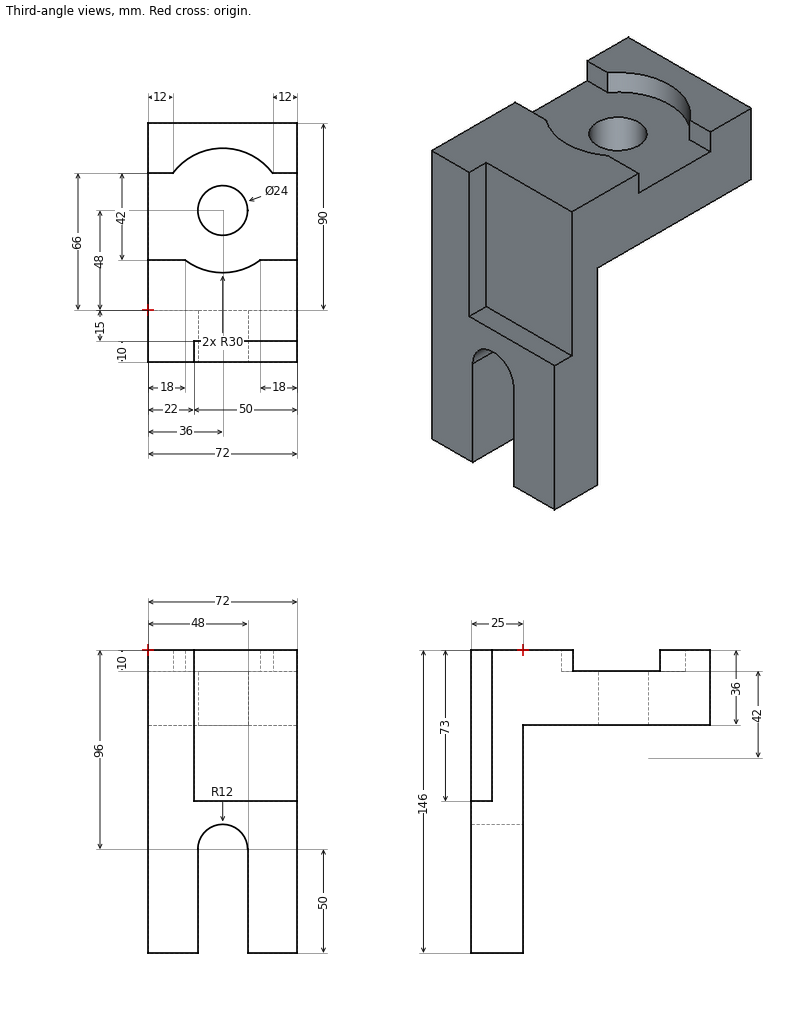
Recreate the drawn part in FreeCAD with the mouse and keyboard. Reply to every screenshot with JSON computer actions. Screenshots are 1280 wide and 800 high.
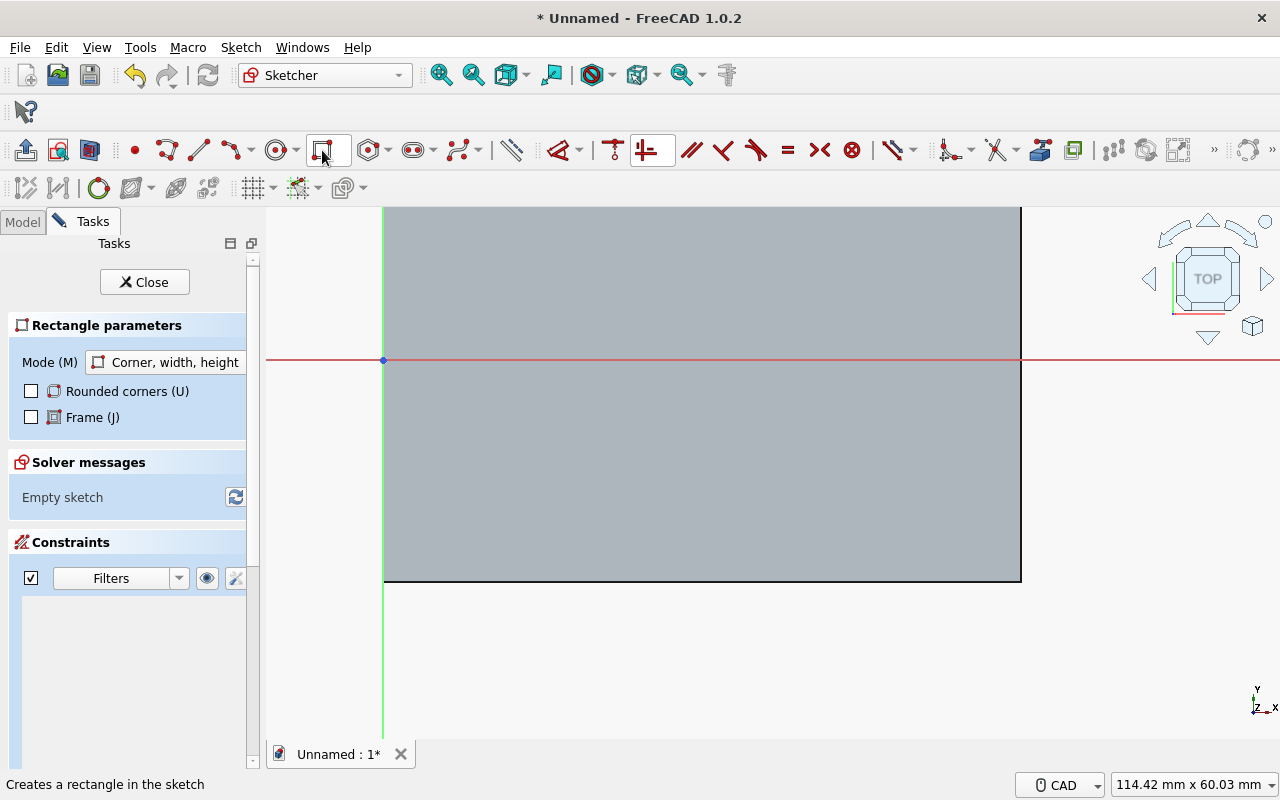
{"action": "left_click", "coordinate": [578, 493]}
{"action": "left_click", "coordinate": [1021, 582]}
{"action": "key", "text": "Escape"}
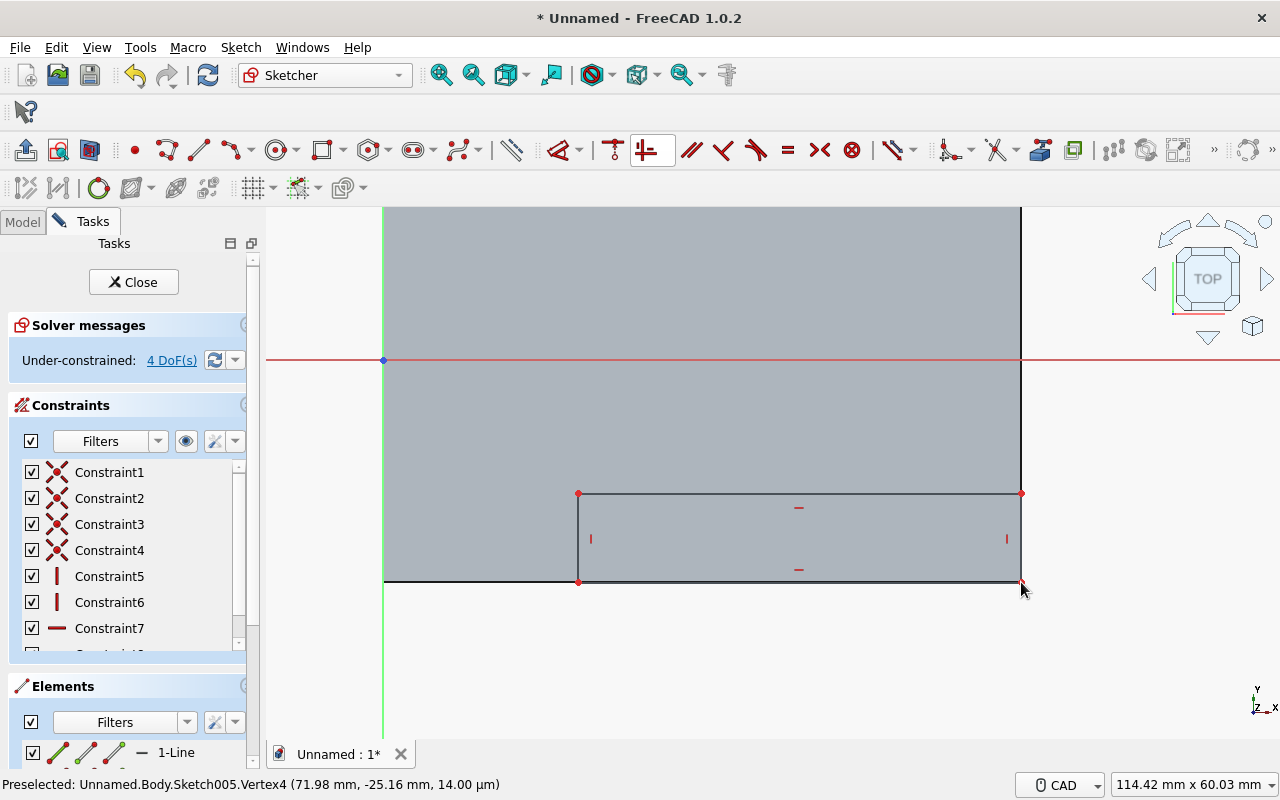
{"action": "left_click", "coordinate": [558, 150]}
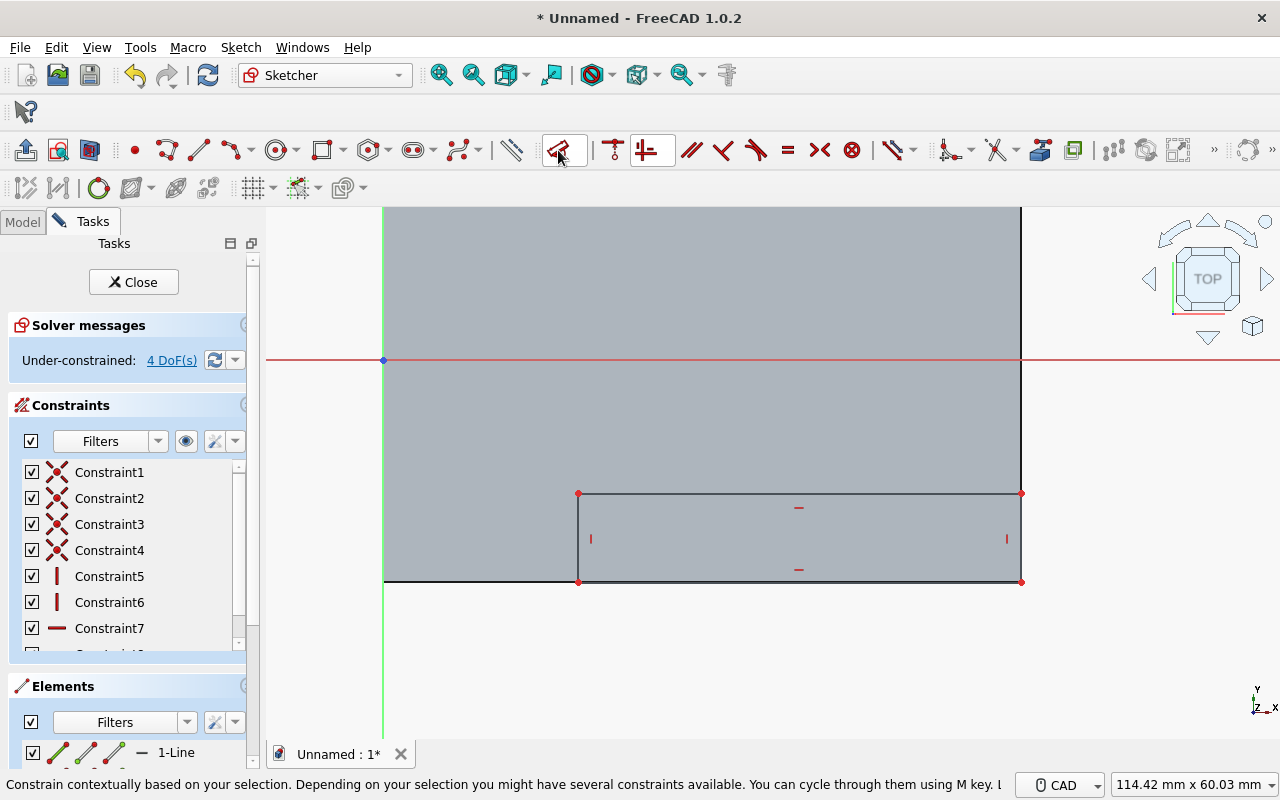
{"action": "left_click", "coordinate": [578, 521]}
{"action": "left_click", "coordinate": [544, 538]}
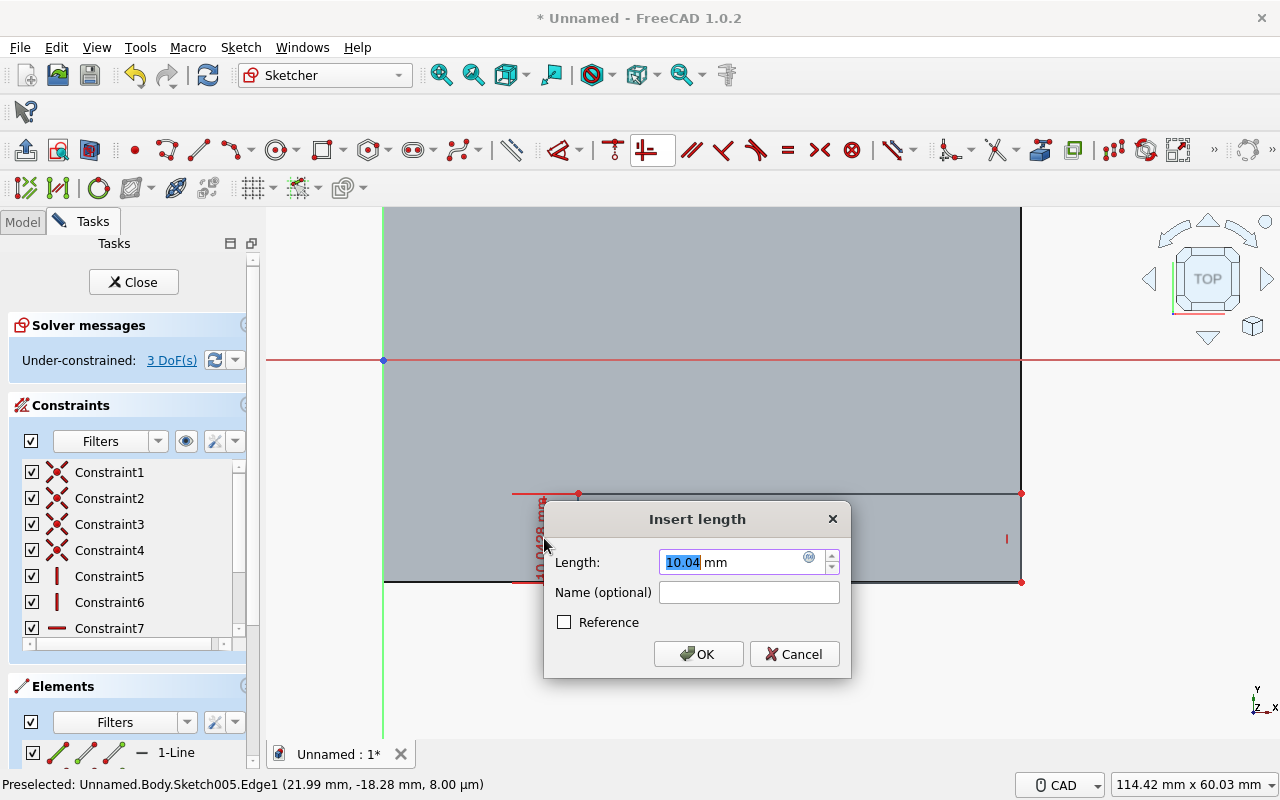
{"action": "type", "text": "10"}
{"action": "key", "text": "Return"}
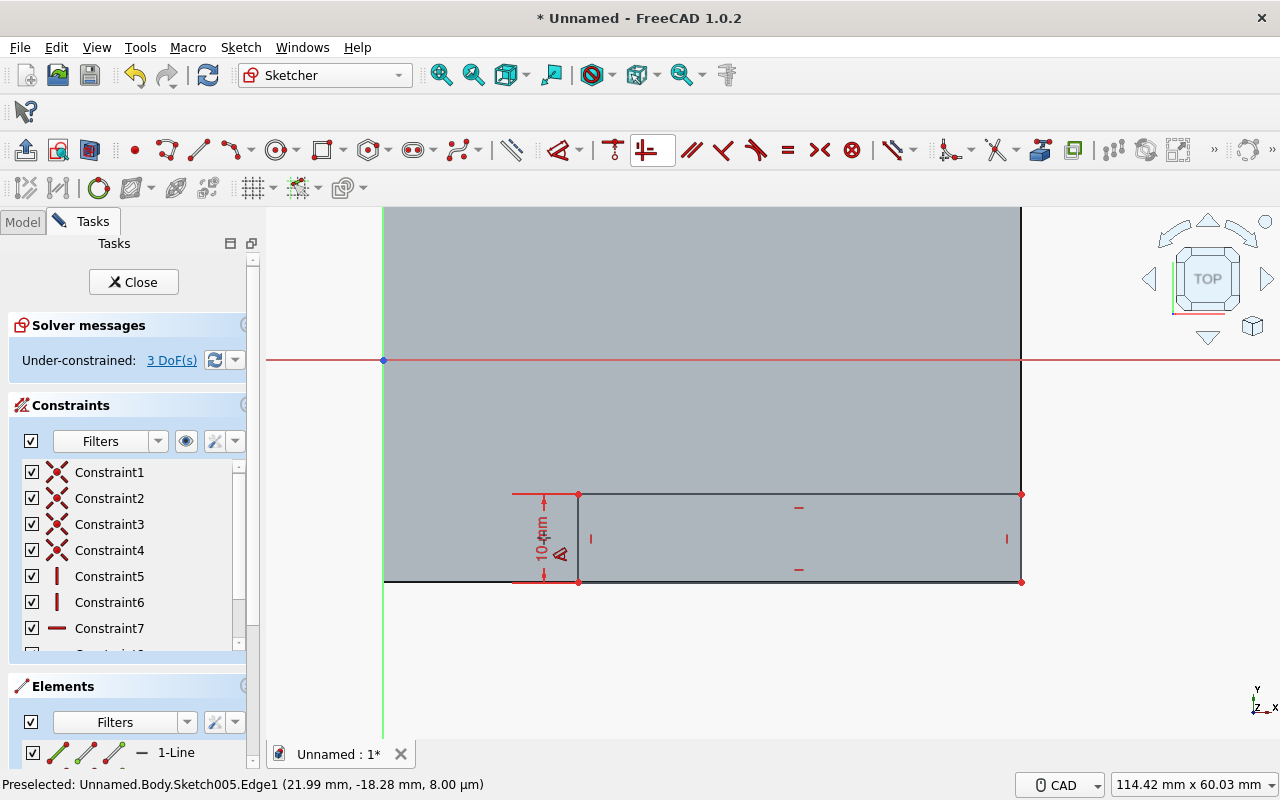
{"action": "left_click", "coordinate": [711, 583]}
{"action": "left_click", "coordinate": [799, 617]}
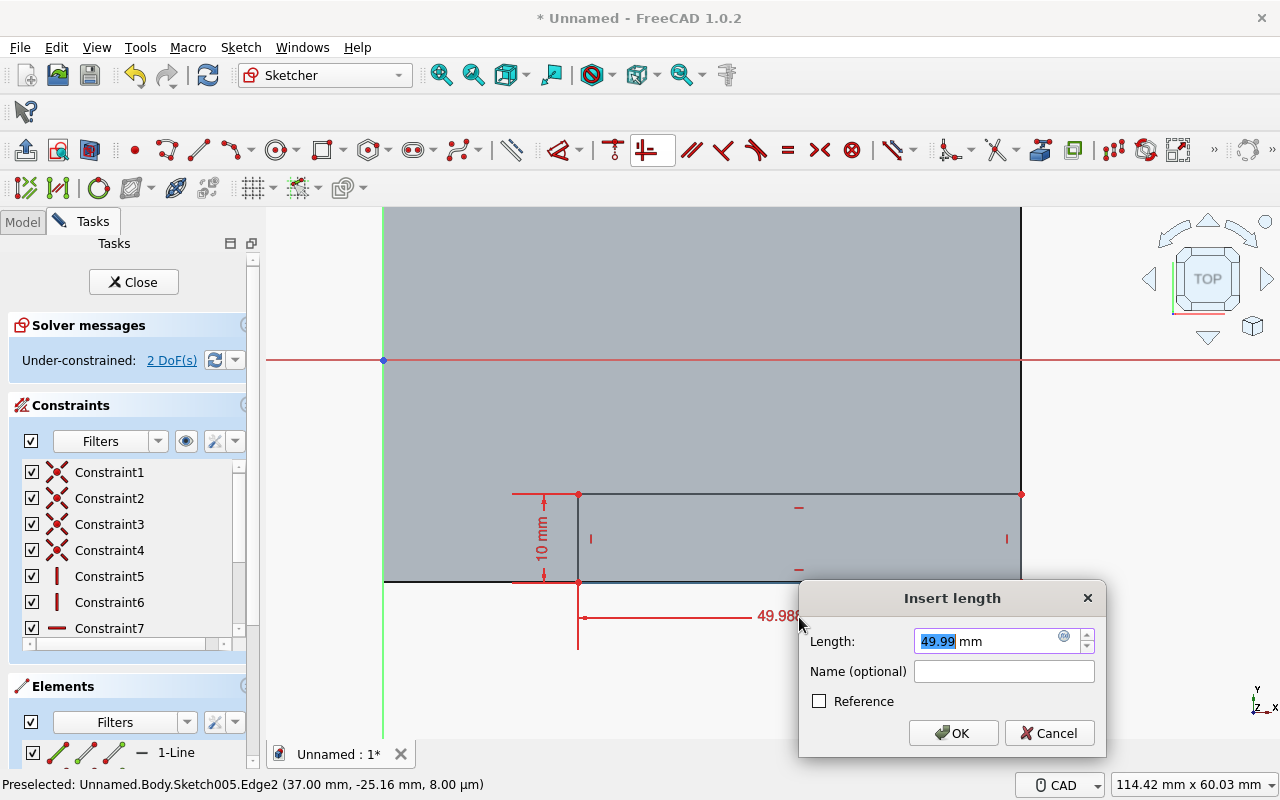
{"action": "type", "text": "50"}
{"action": "key", "text": "Return"}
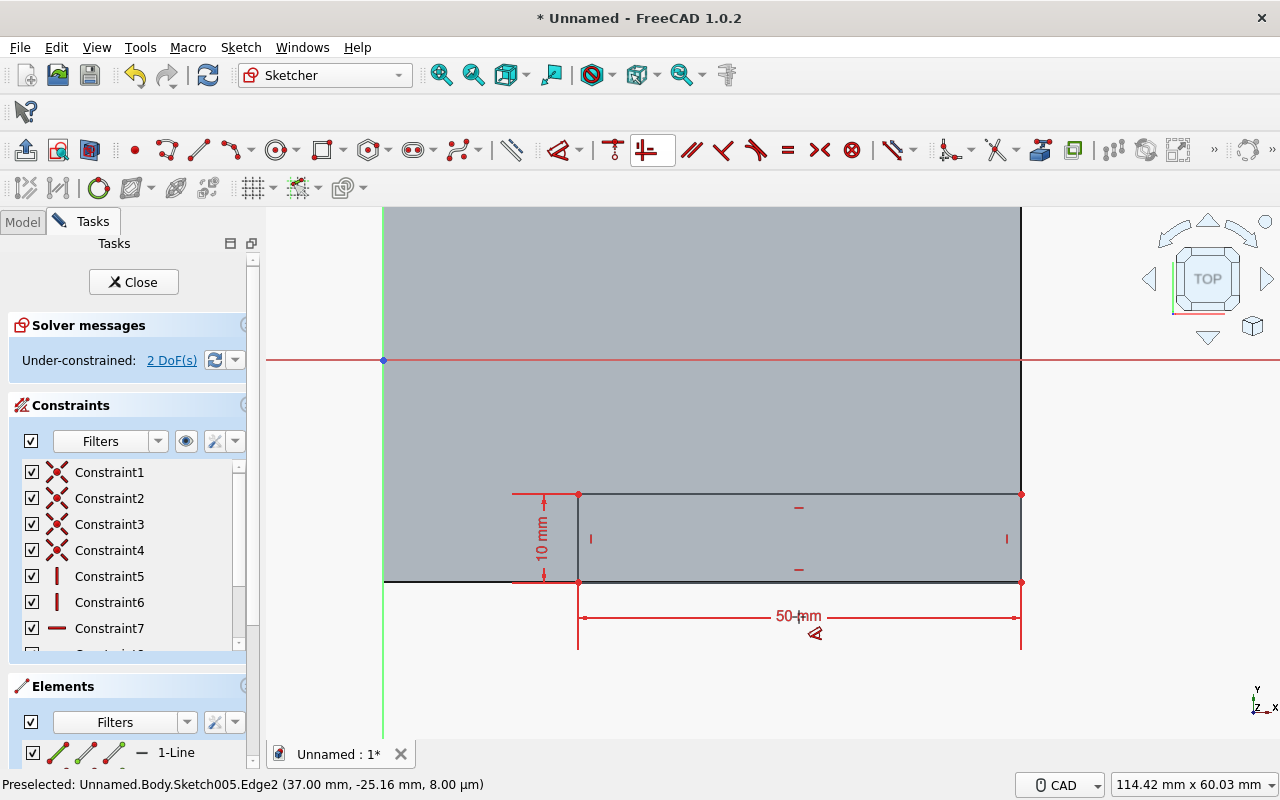
{"action": "left_click", "coordinate": [578, 494]}
{"action": "left_click", "coordinate": [481, 326]}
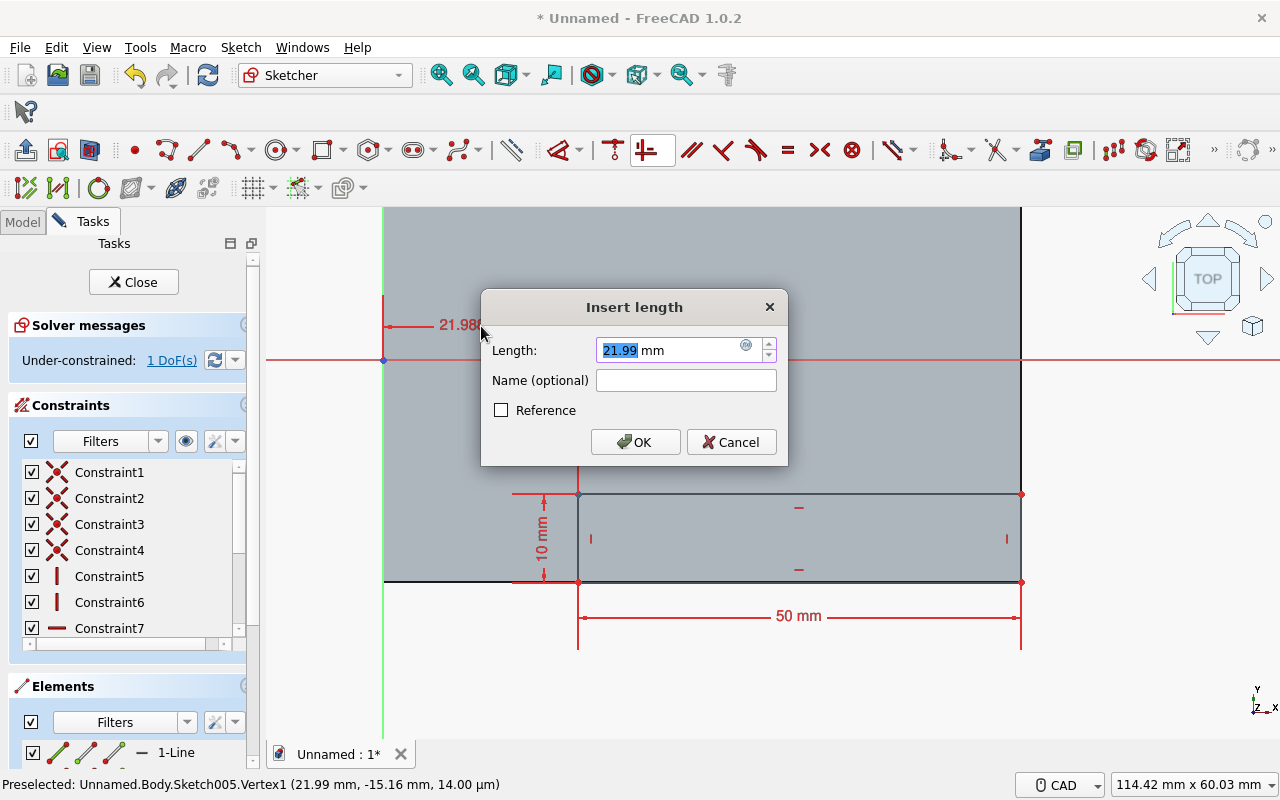
{"action": "type", "text": "22"}
{"action": "key", "text": "Return"}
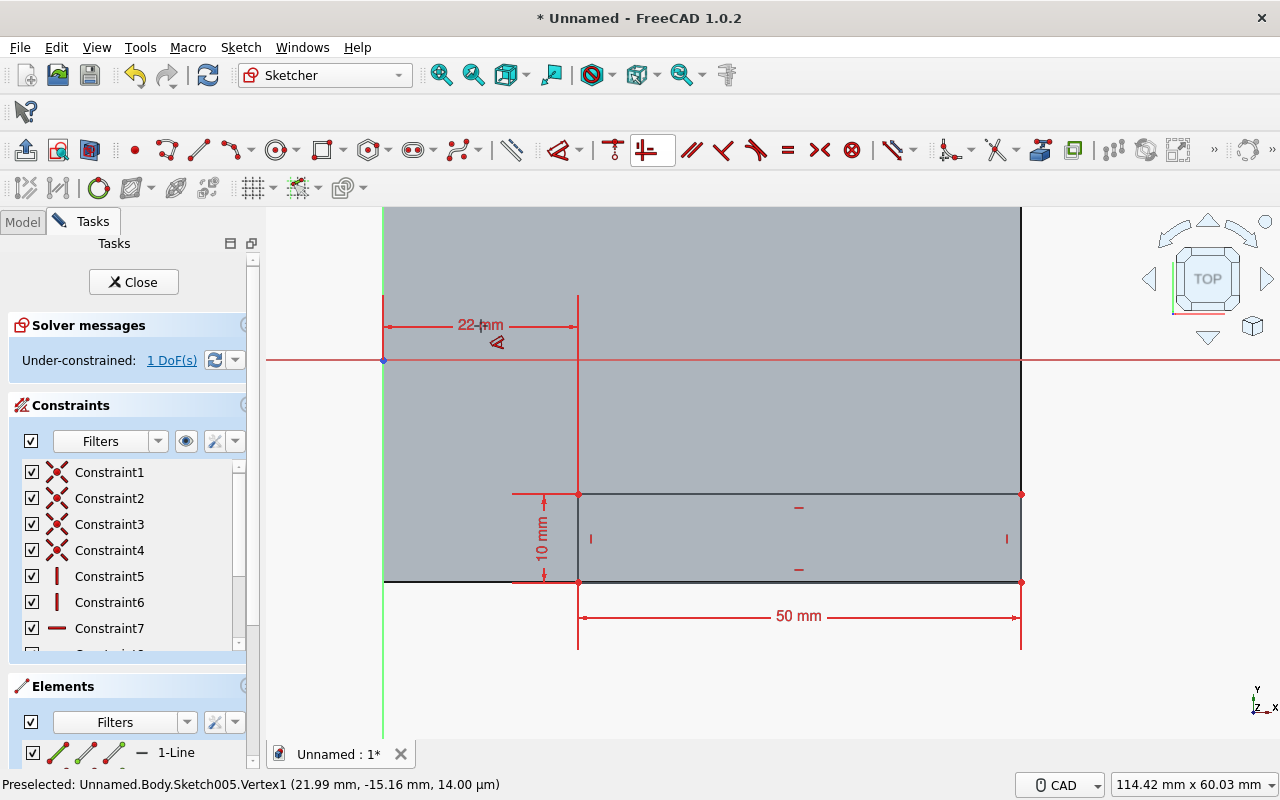
{"action": "left_click", "coordinate": [578, 494]}
{"action": "left_click", "coordinate": [349, 427]}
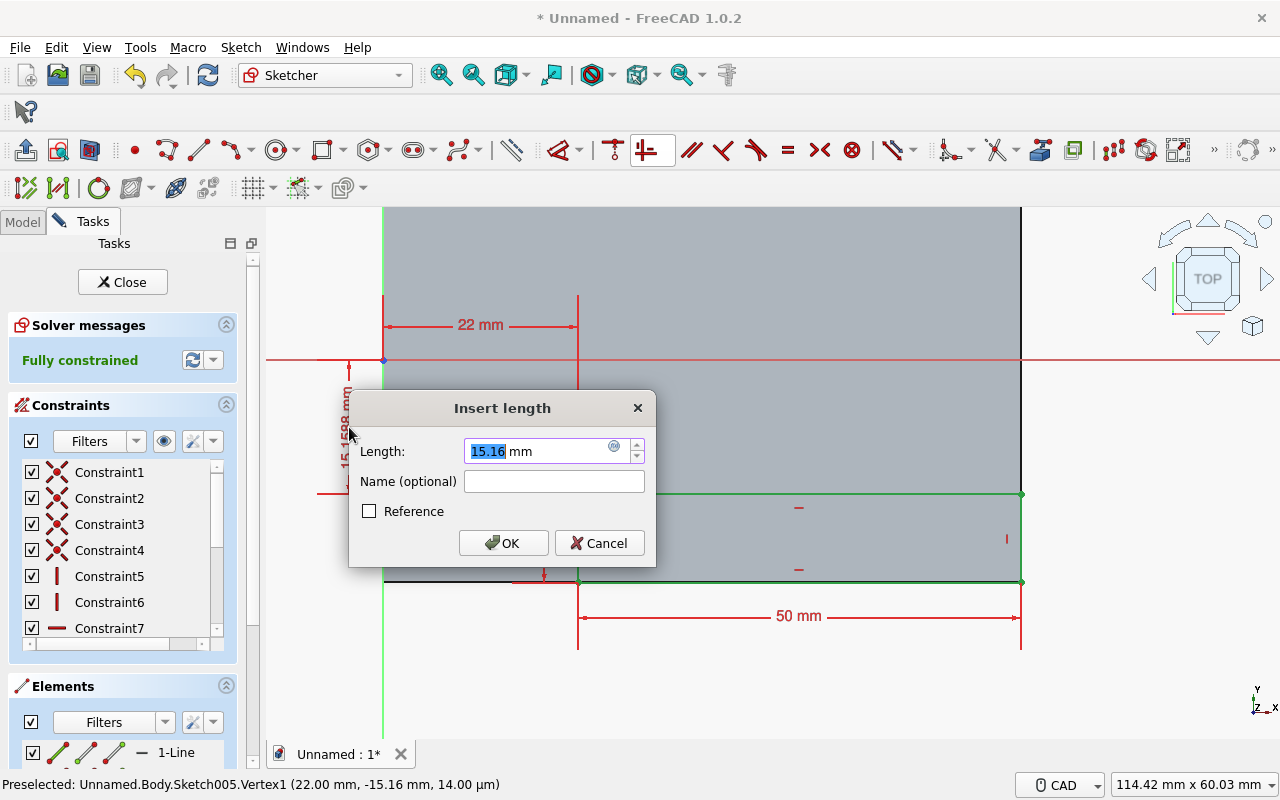
{"action": "type", "text": "15"}
{"action": "key", "text": "Return"}
{"action": "key", "text": "Escape"}